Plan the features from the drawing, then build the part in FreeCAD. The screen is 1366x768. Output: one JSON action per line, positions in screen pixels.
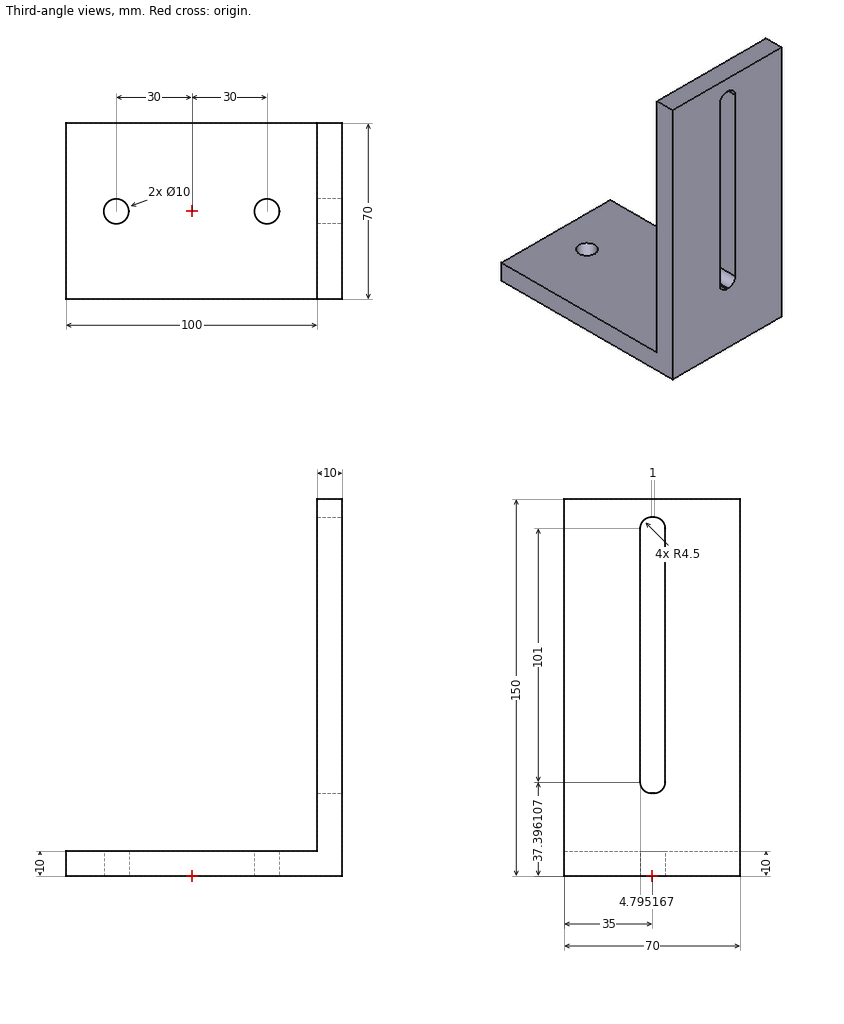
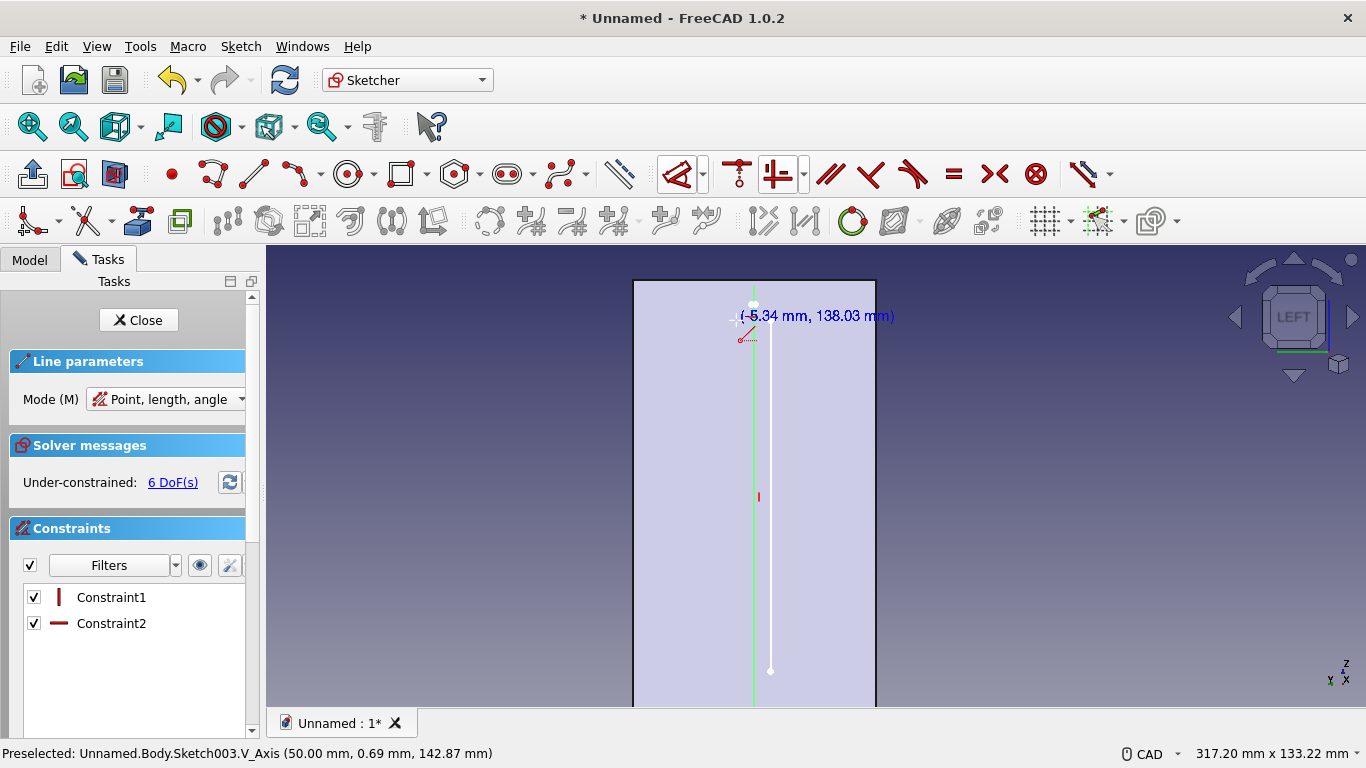
{"action": "left_click", "coordinate": [736, 320]}
{"action": "left_click", "coordinate": [736, 670]}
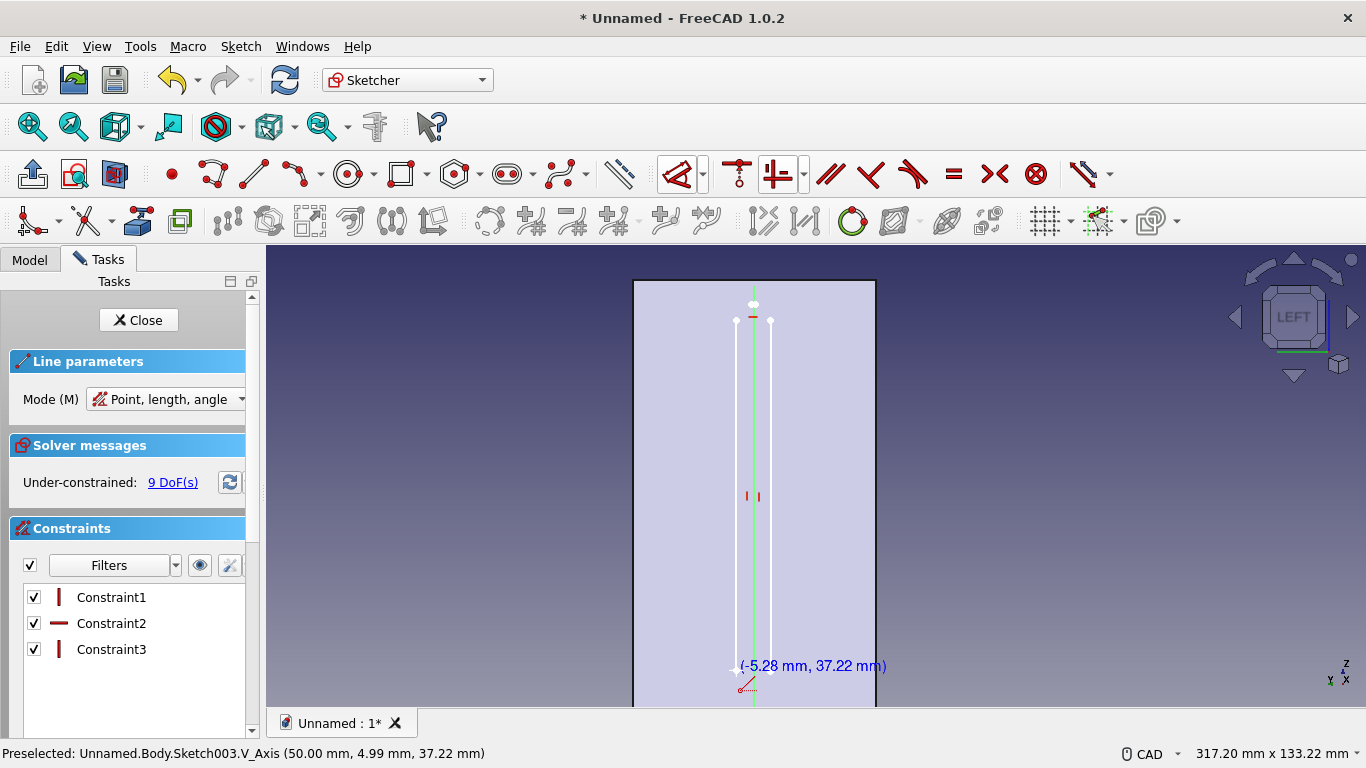
{"action": "scroll", "coordinate": [740, 383], "scroll_direction": "down", "scroll_amount": 3}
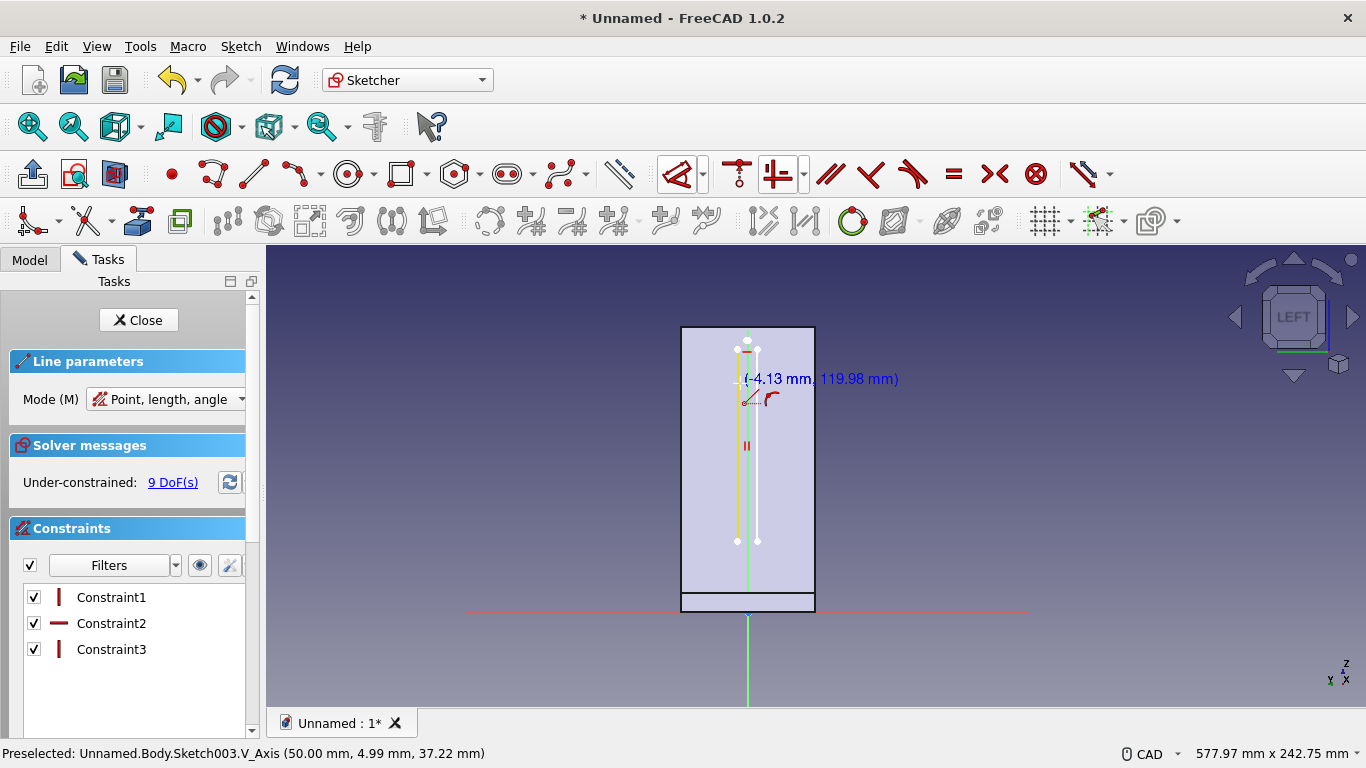
{"action": "scroll", "coordinate": [747, 549], "scroll_direction": "up", "scroll_amount": 13}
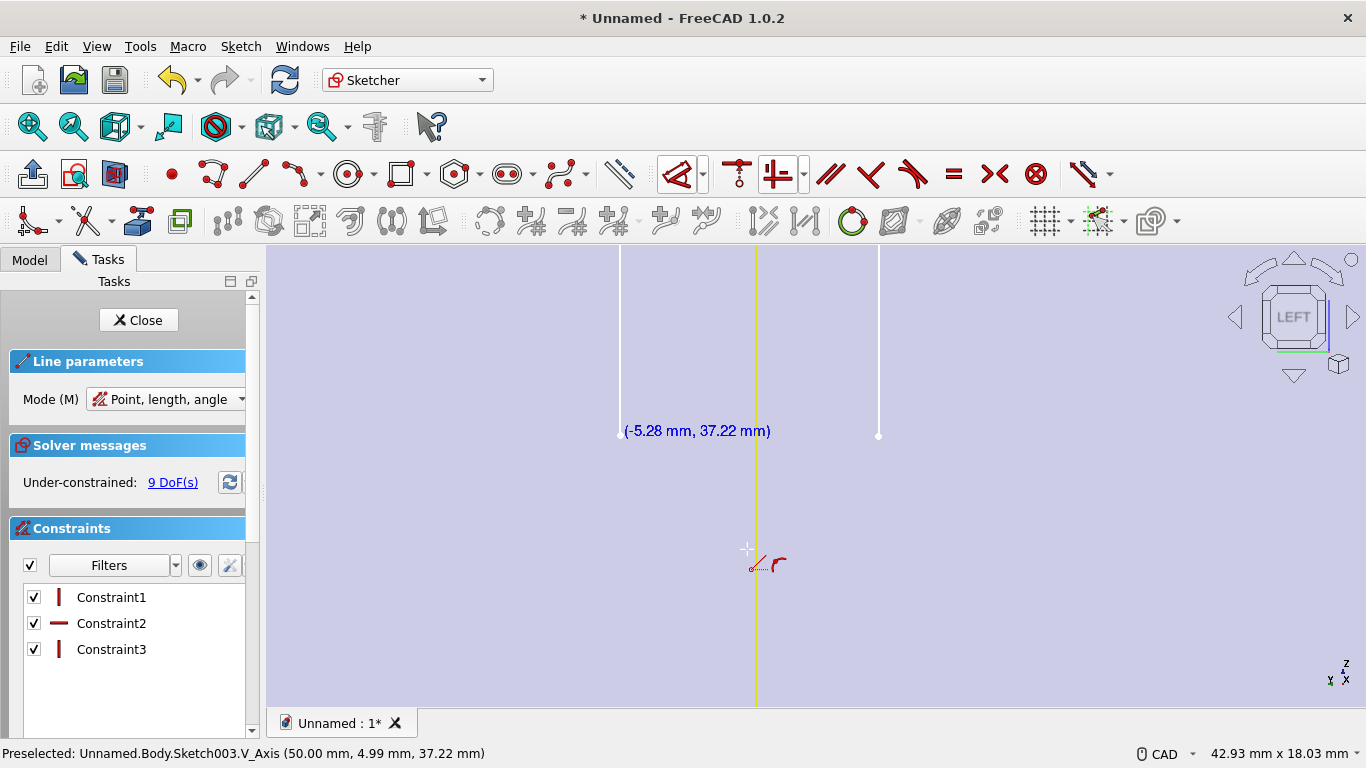
{"action": "left_click", "coordinate": [738, 546]}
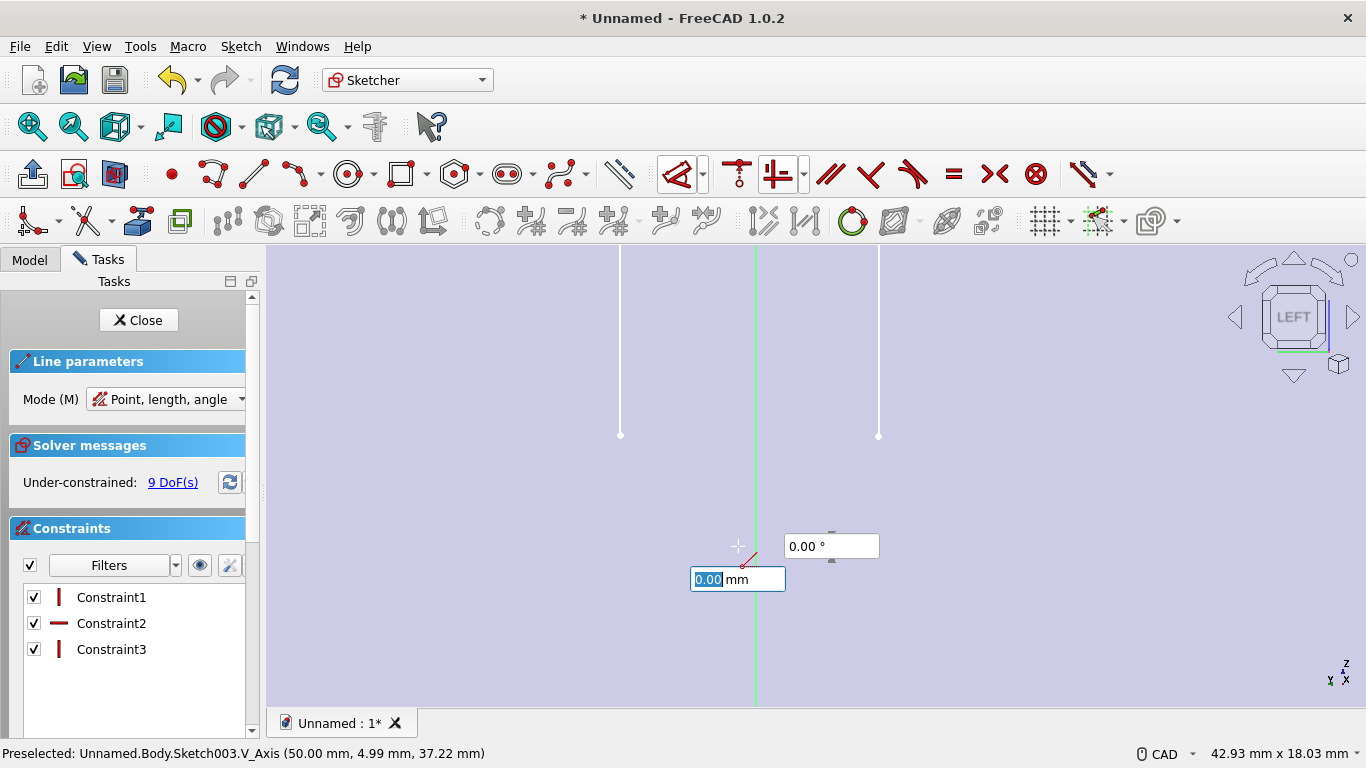
{"action": "scroll", "coordinate": [763, 546], "scroll_direction": "up", "scroll_amount": 4}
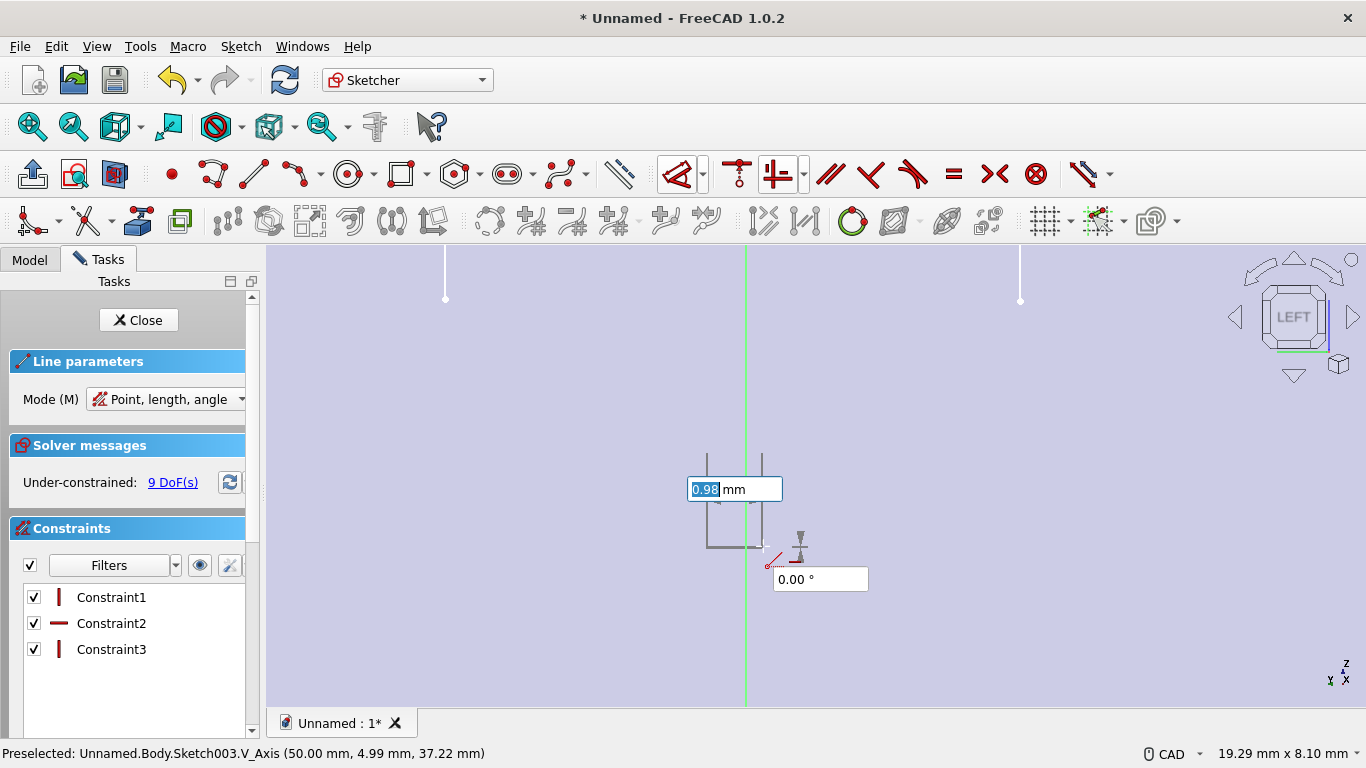
{"action": "left_click", "coordinate": [763, 545]}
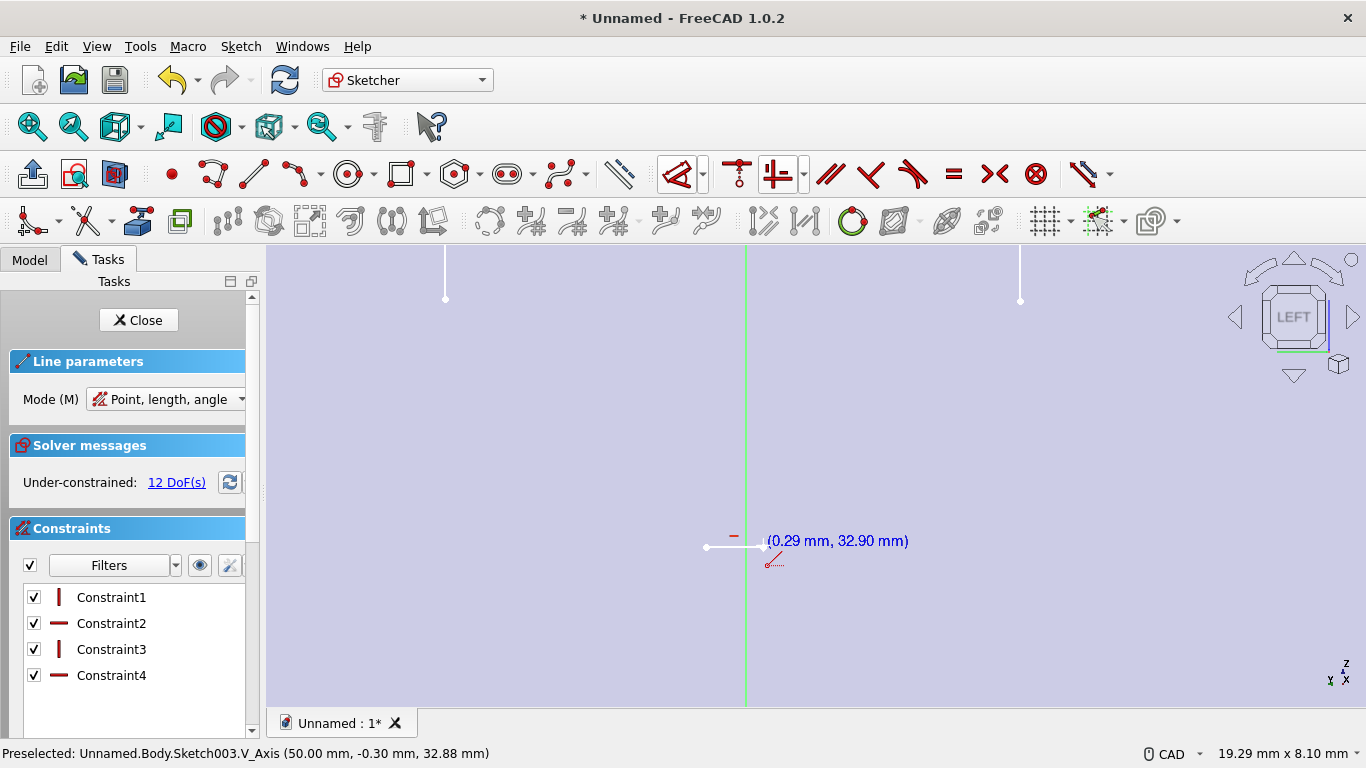
{"action": "left_click", "coordinate": [294, 174]}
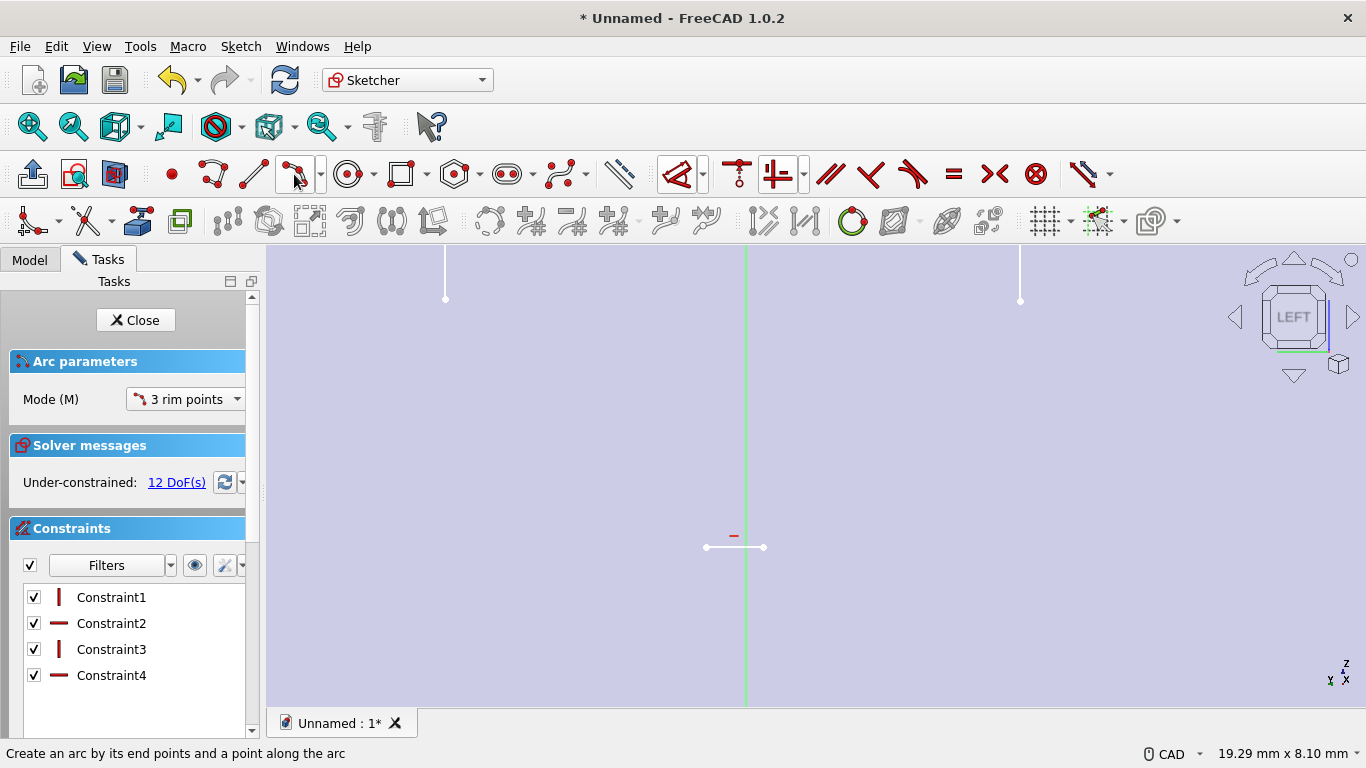
{"action": "scroll", "coordinate": [748, 566], "scroll_direction": "down", "scroll_amount": 16}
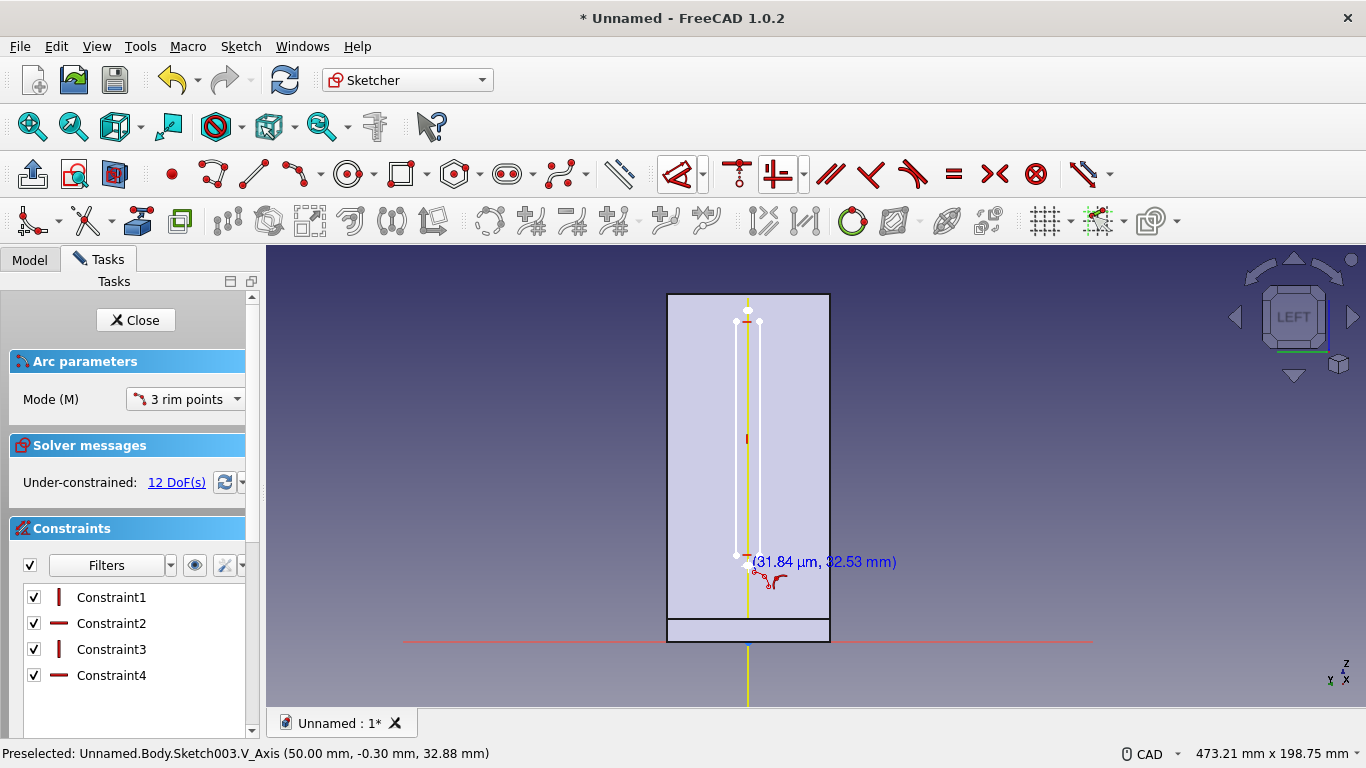
{"action": "scroll", "coordinate": [759, 321], "scroll_direction": "up", "scroll_amount": 2}